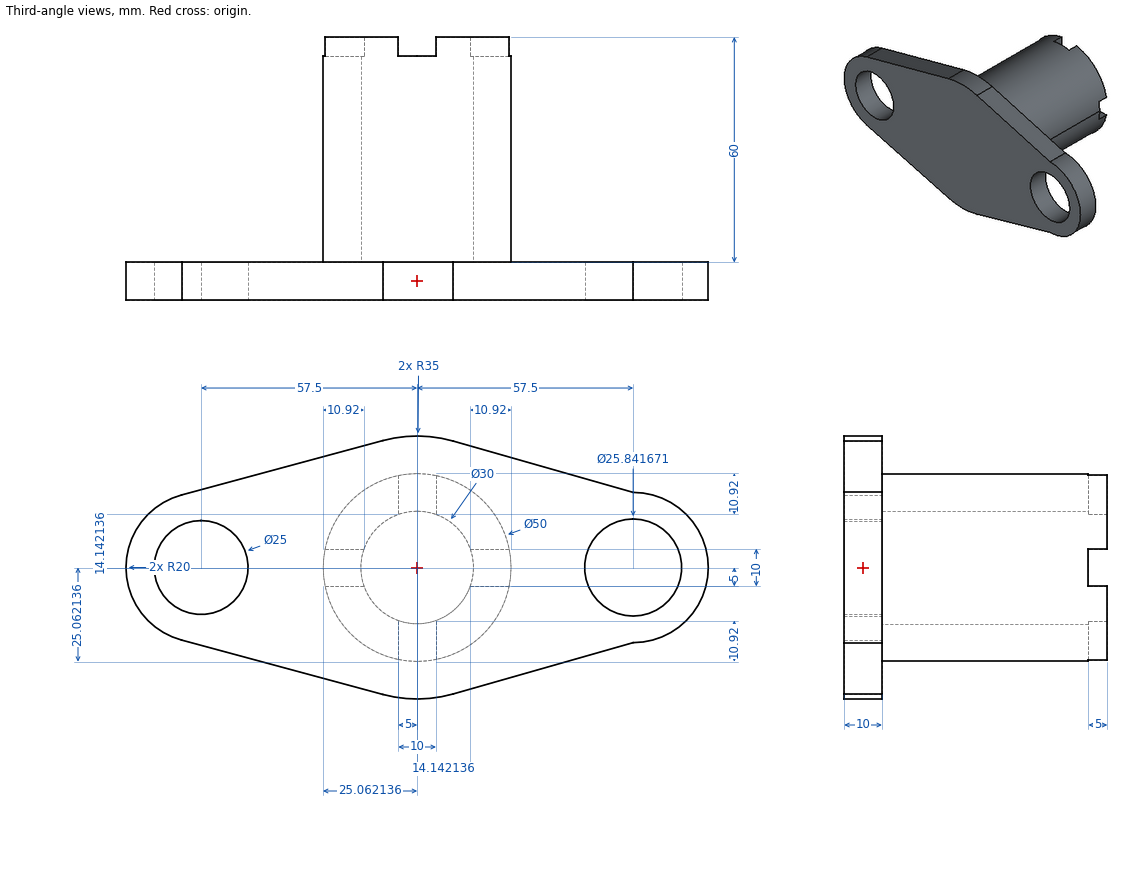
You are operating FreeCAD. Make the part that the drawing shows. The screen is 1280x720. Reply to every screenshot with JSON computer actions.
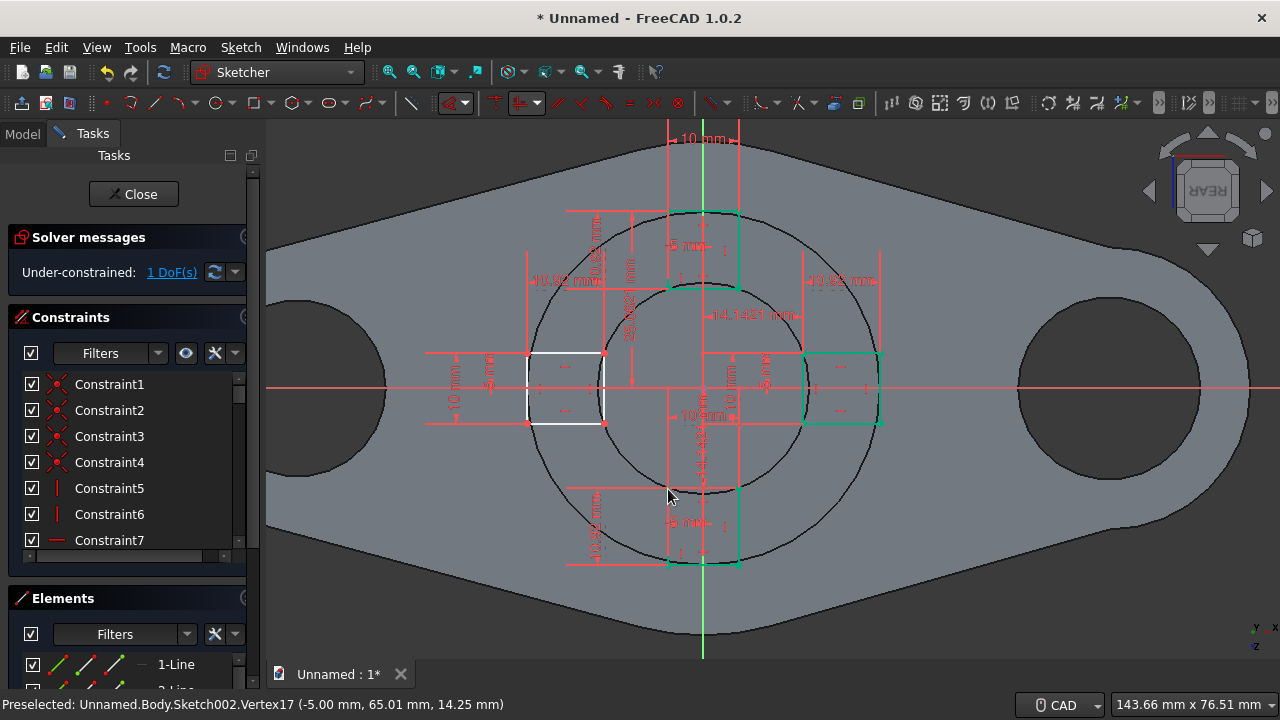
{"action": "left_click", "coordinate": [527, 353]}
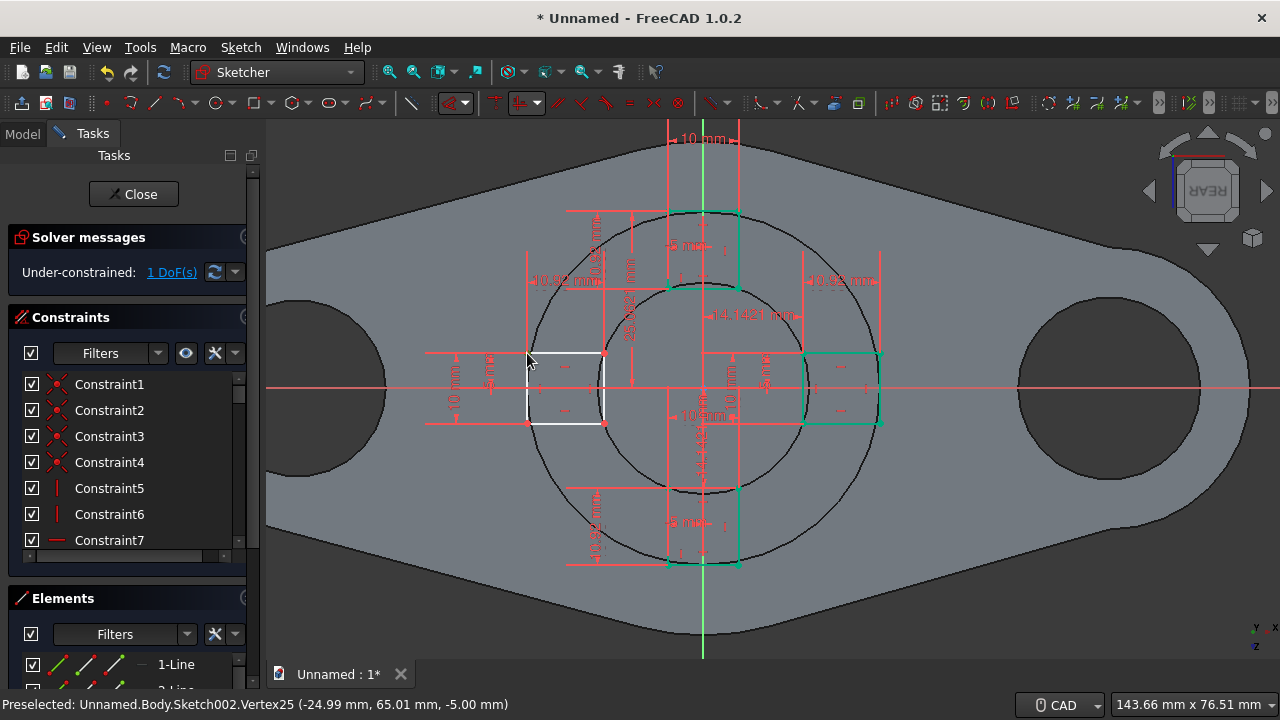
{"action": "left_click", "coordinate": [468, 104]}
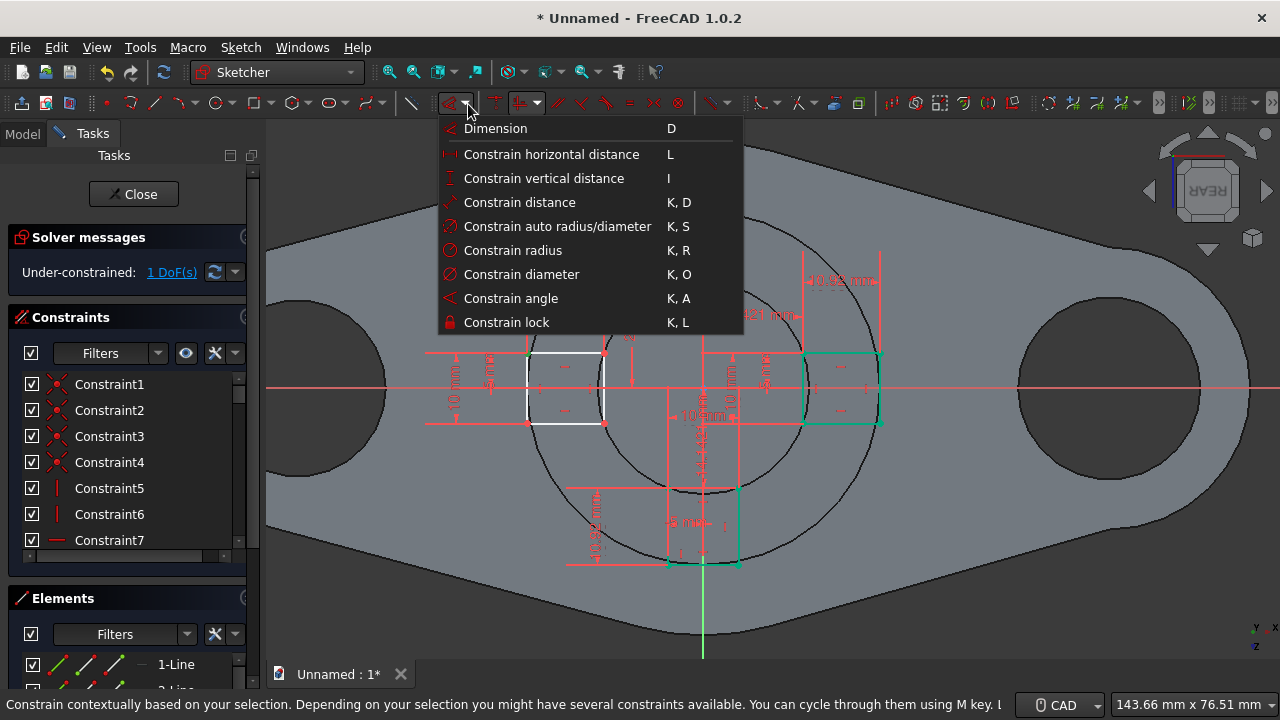
{"action": "left_click", "coordinate": [591, 154]}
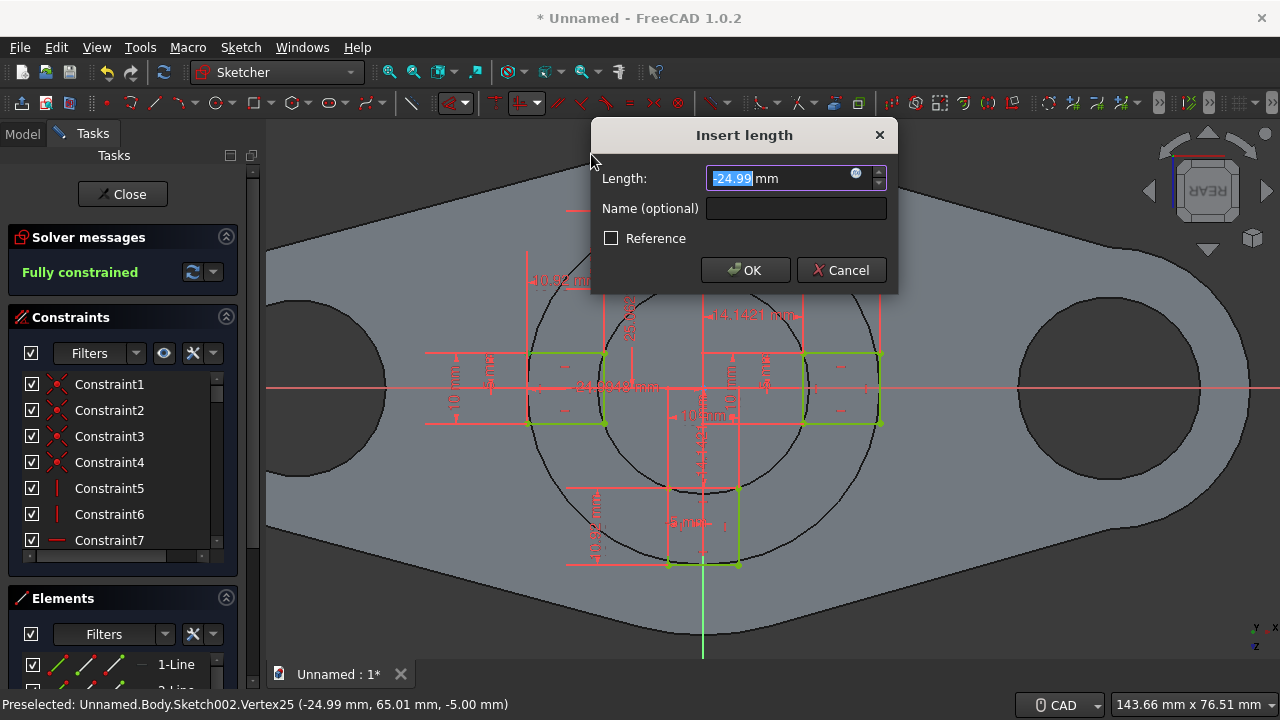
{"action": "type", "text": "-25.062136"}
{"action": "key", "text": "Return"}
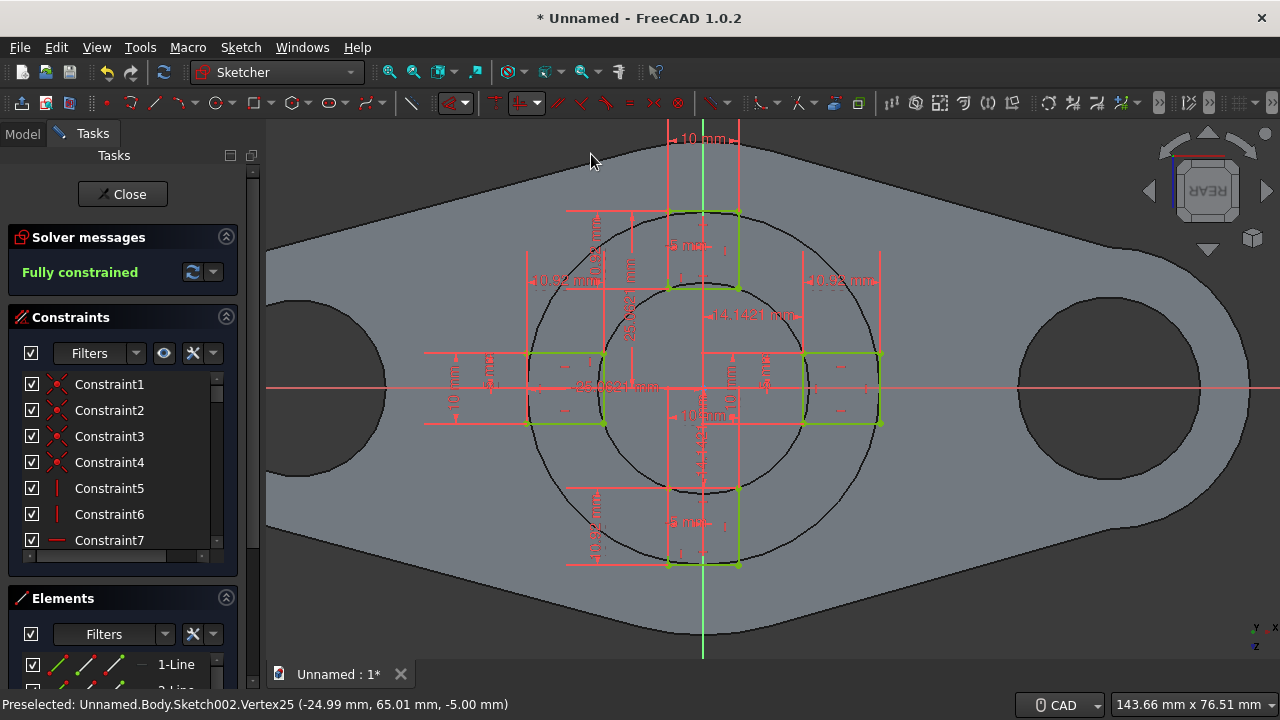
{"action": "left_click", "coordinate": [123, 194]}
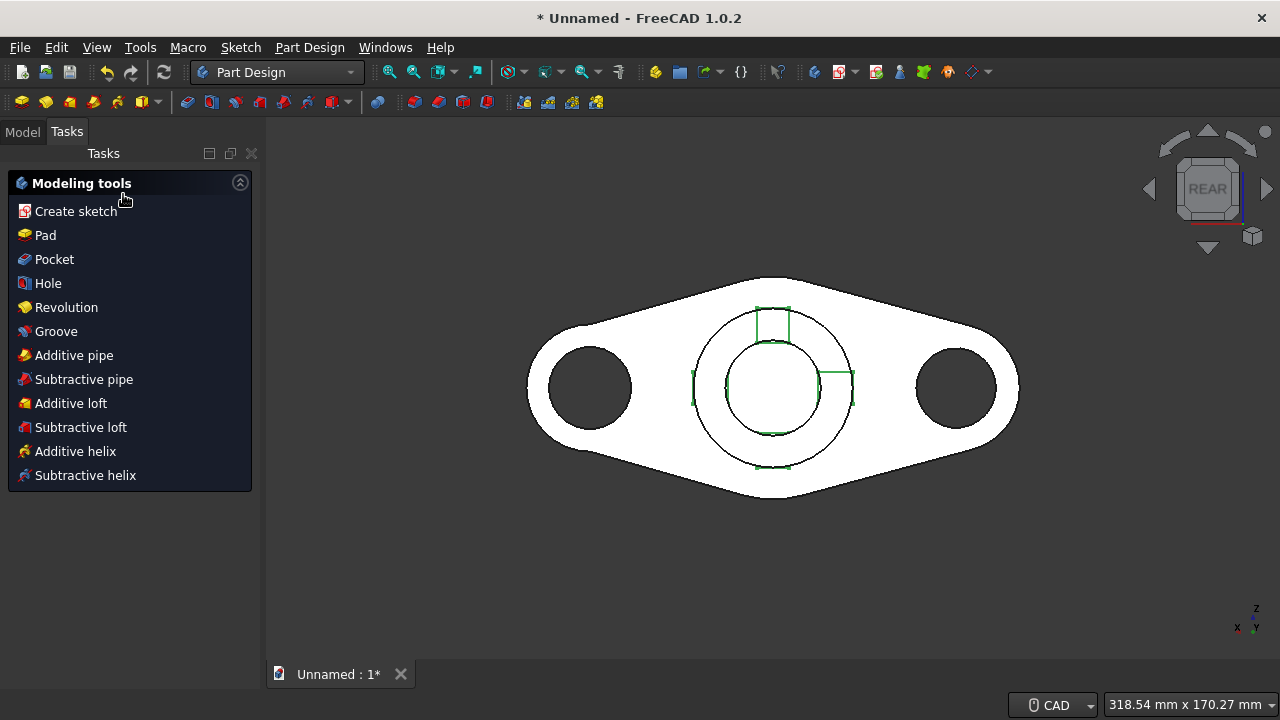
{"action": "left_click", "coordinate": [188, 102]}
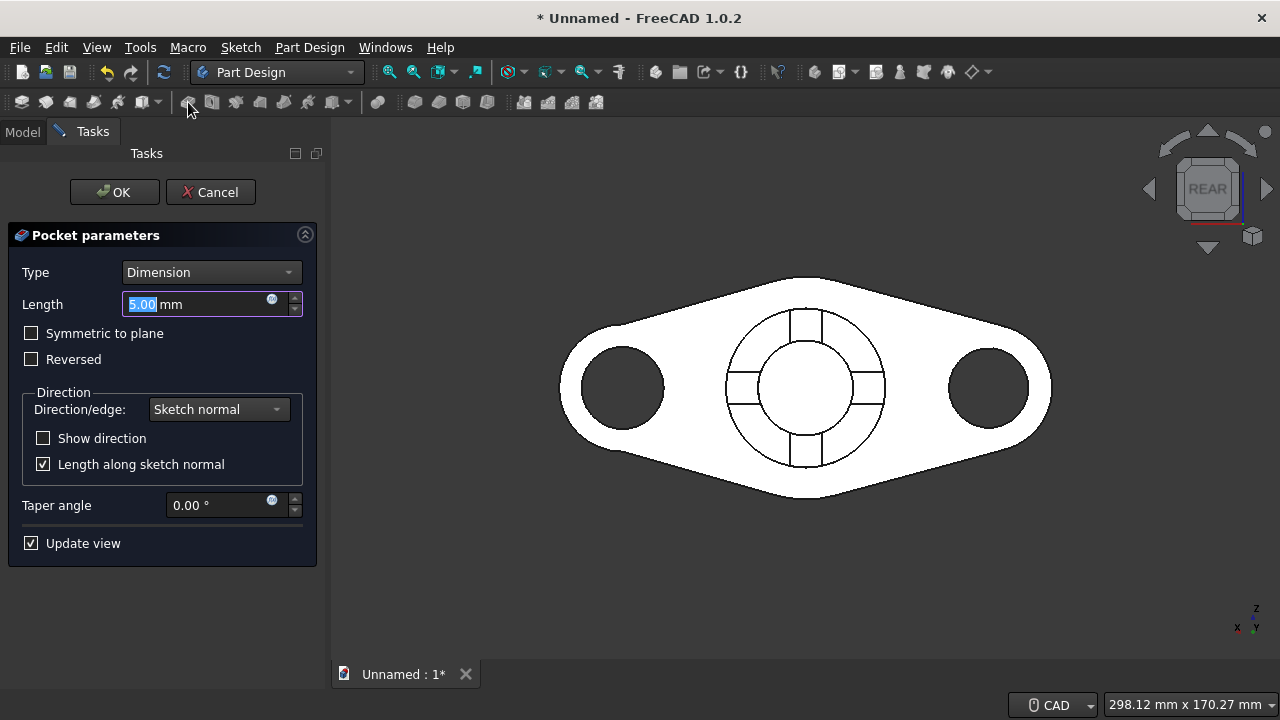
{"action": "type", "text": "5"}
{"action": "key", "text": "Tab"}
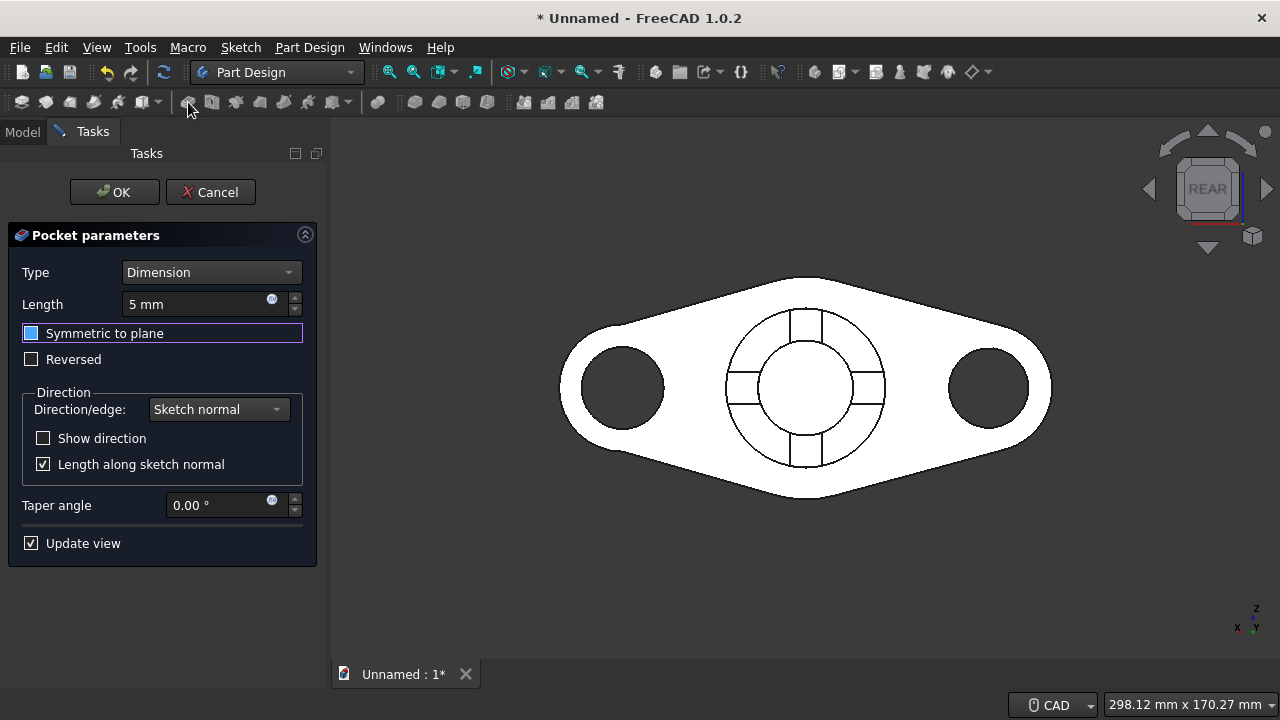
{"action": "left_click", "coordinate": [115, 192]}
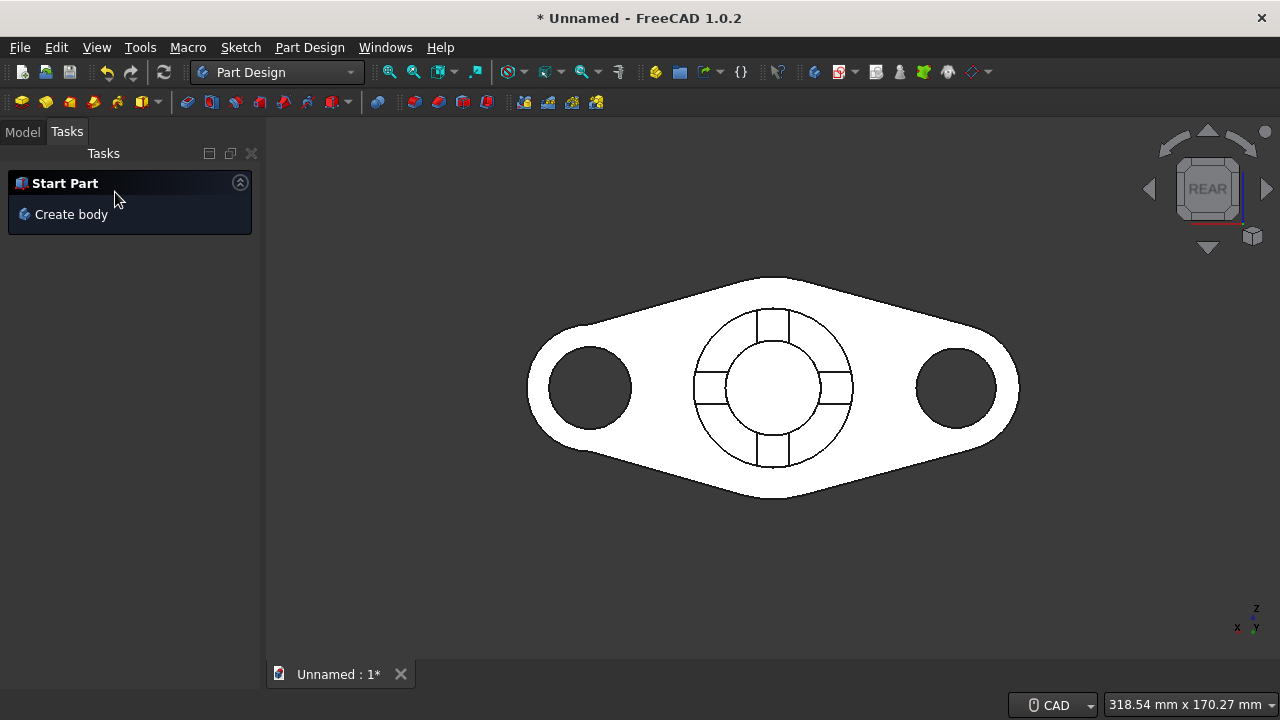
{"action": "key", "text": "0"}